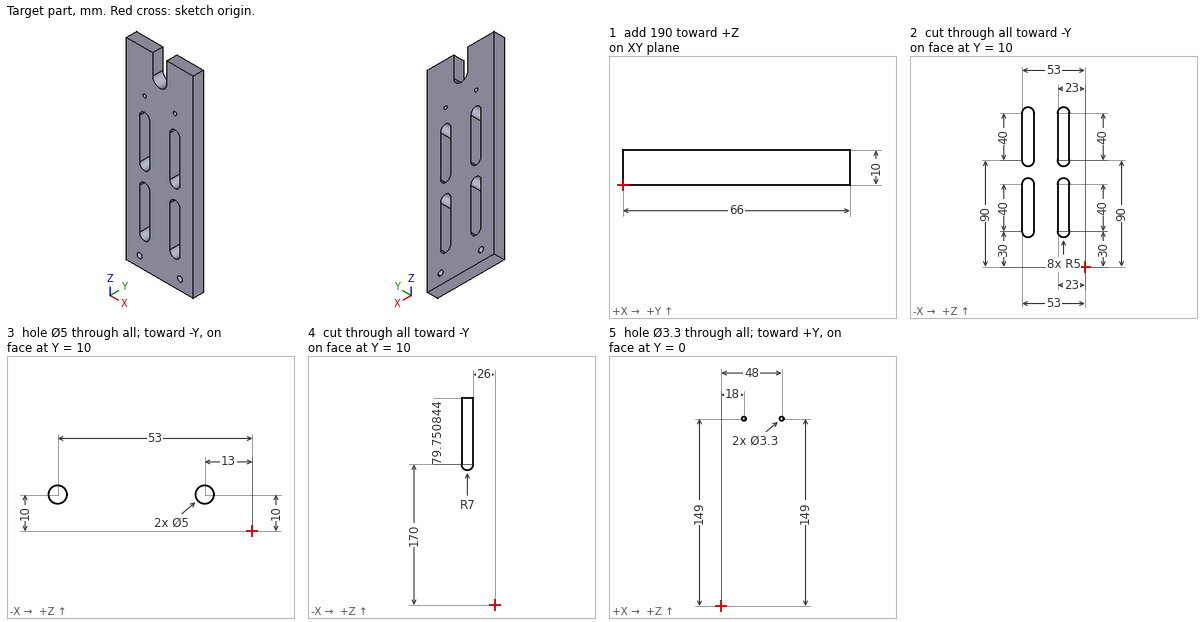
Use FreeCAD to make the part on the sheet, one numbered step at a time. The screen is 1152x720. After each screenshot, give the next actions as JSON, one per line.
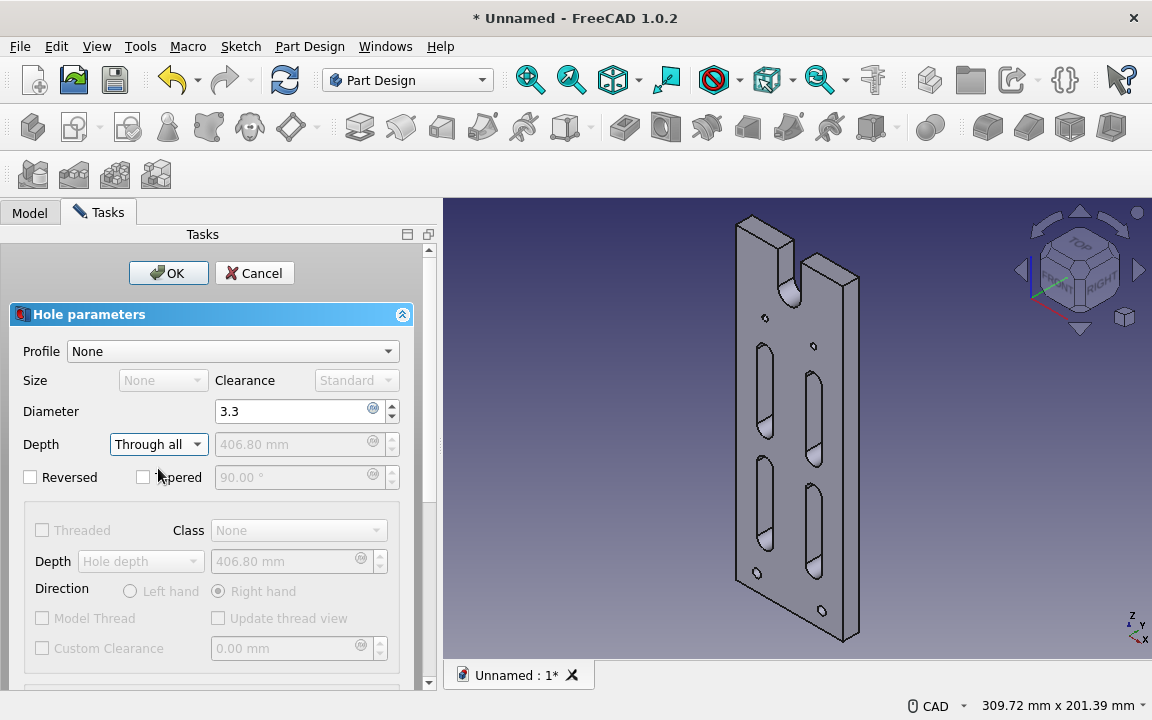
{"action": "left_click", "coordinate": [169, 273]}